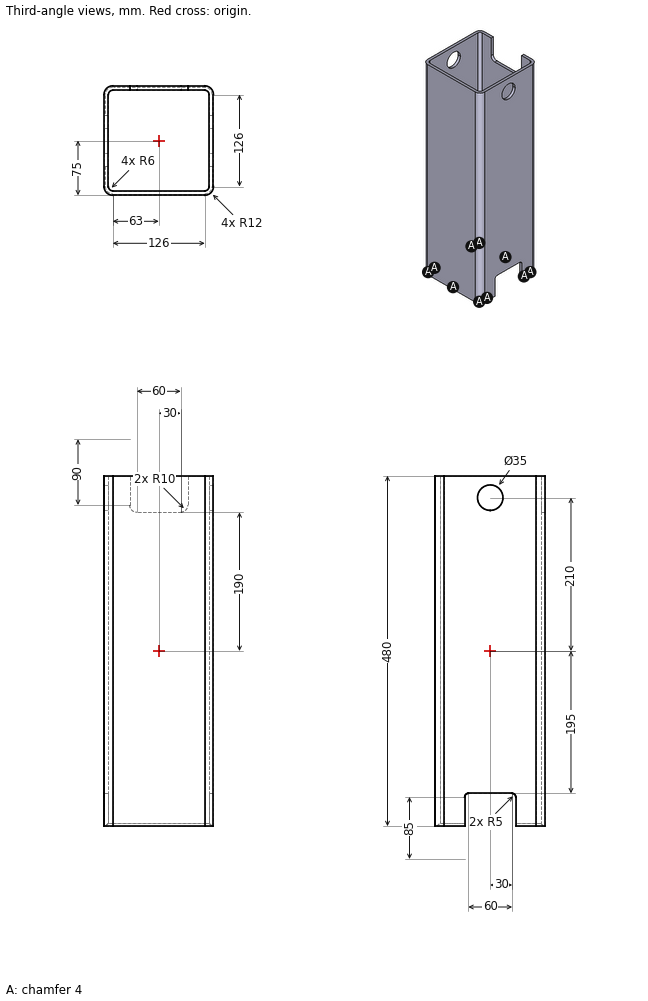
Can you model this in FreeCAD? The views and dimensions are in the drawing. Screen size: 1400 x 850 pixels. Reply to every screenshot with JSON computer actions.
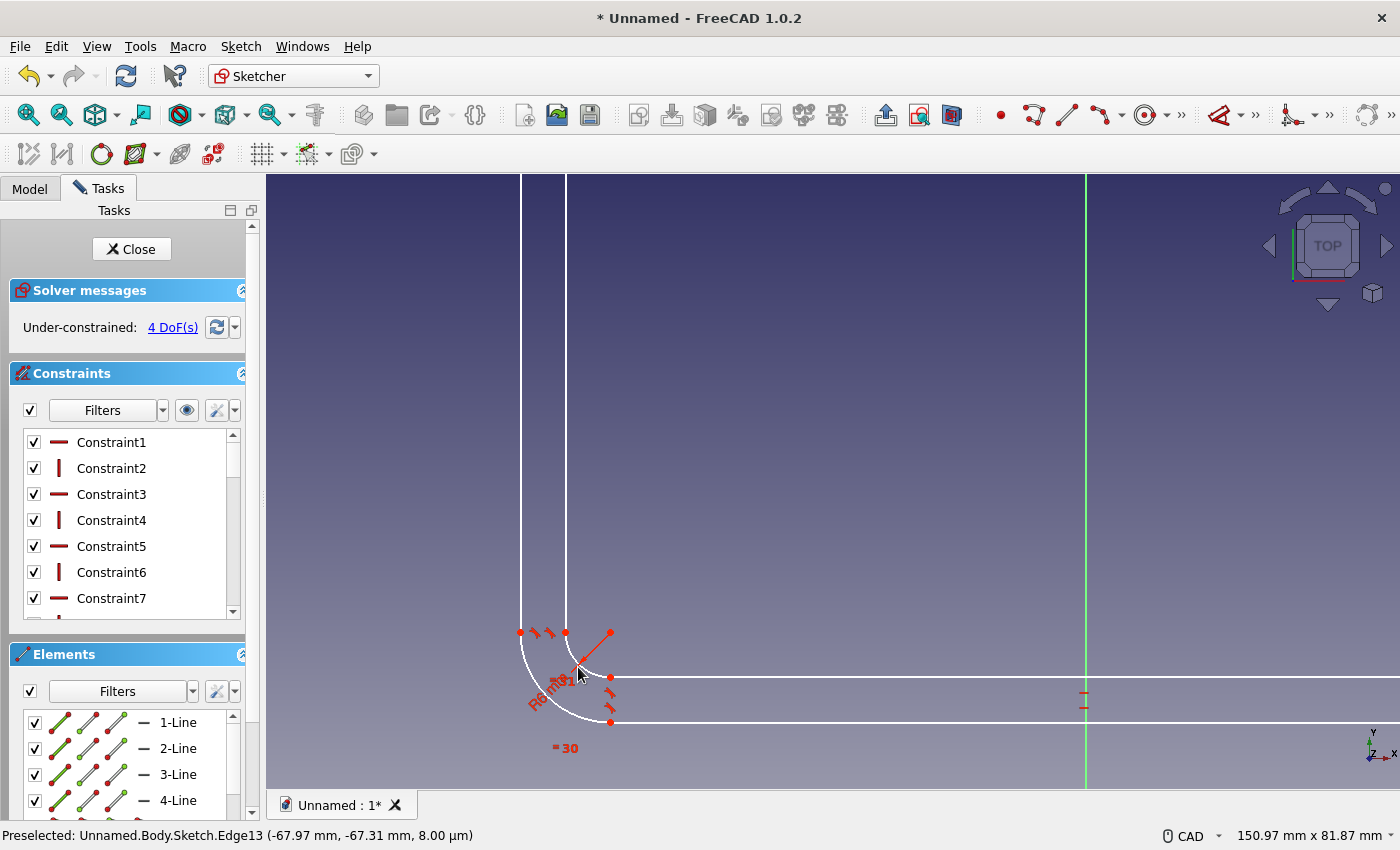
{"action": "left_click", "coordinate": [895, 723]}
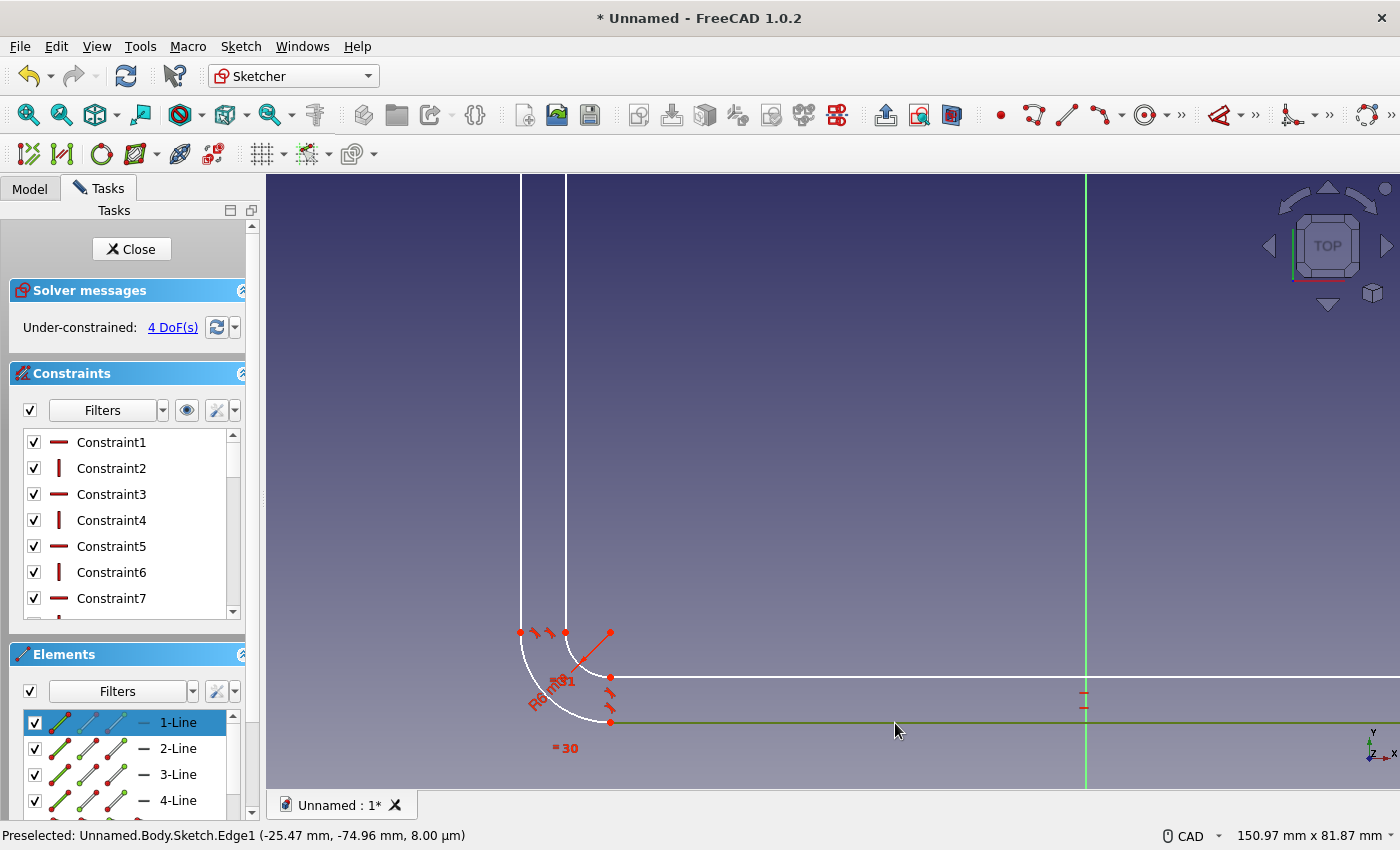
{"action": "key", "text": "l"}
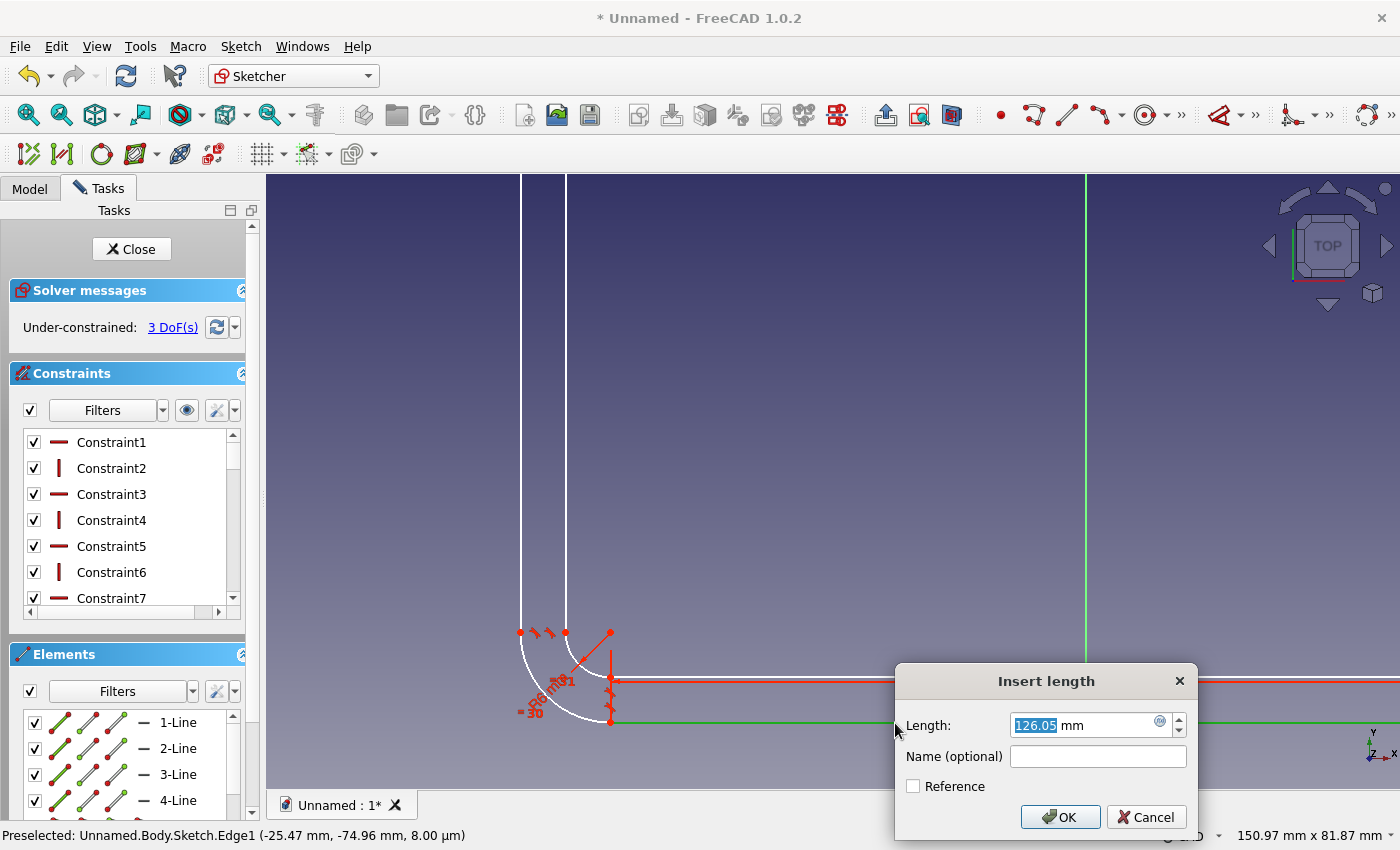
{"action": "type", "text": "126"}
{"action": "key", "text": "Return"}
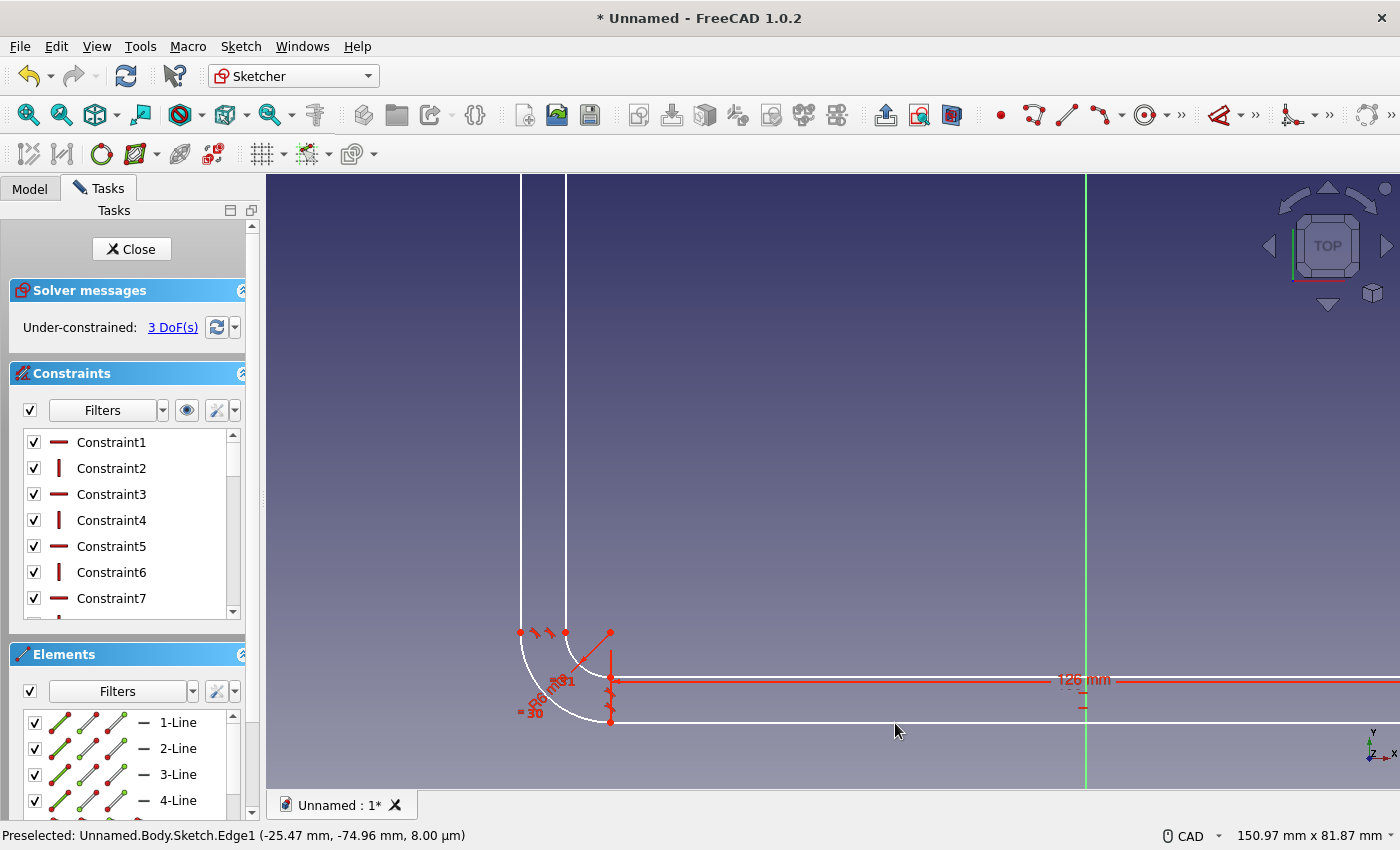
{"action": "scroll", "coordinate": [577, 669], "scroll_direction": "down", "scroll_amount": 5}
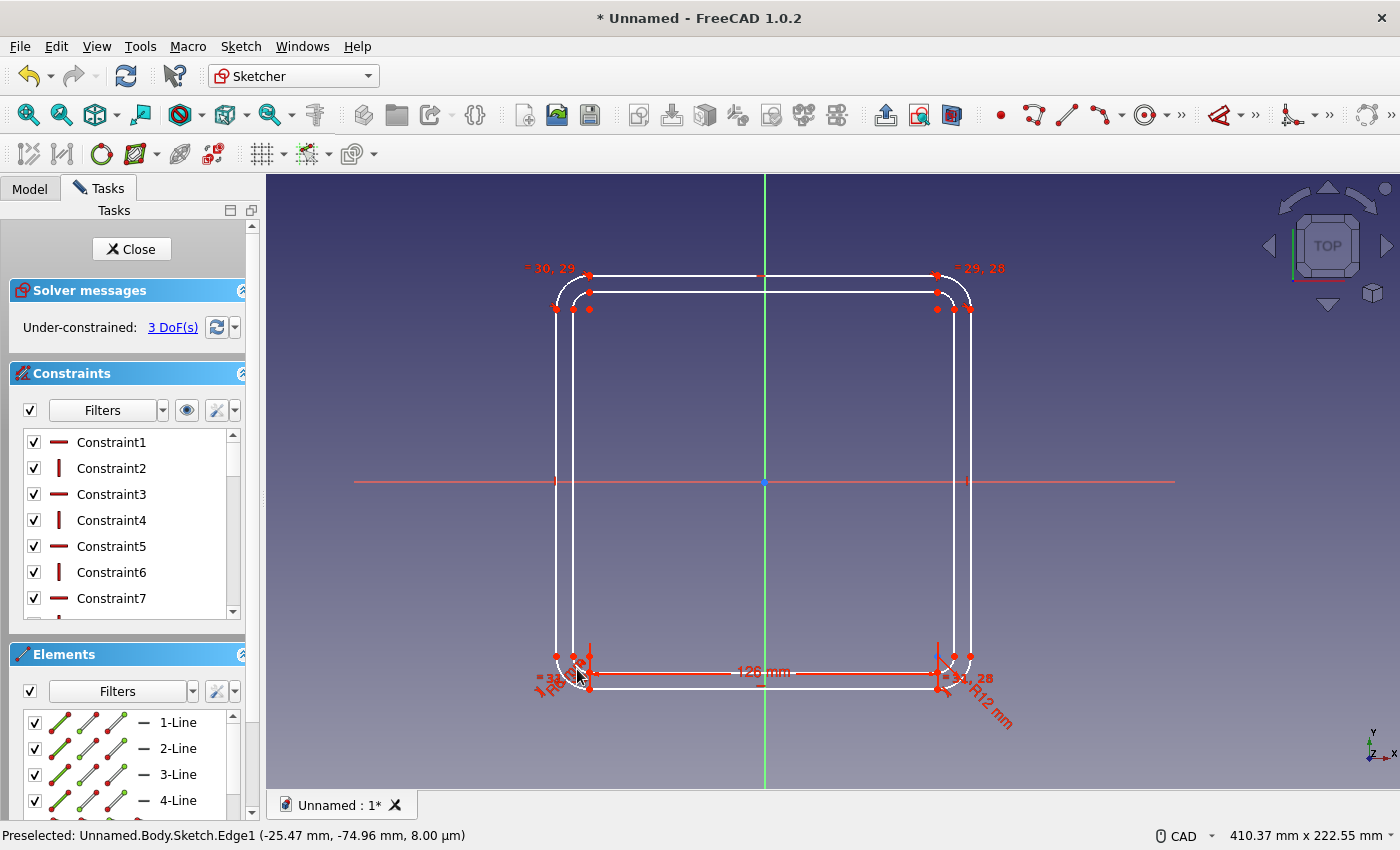
{"action": "left_click", "coordinate": [971, 552]}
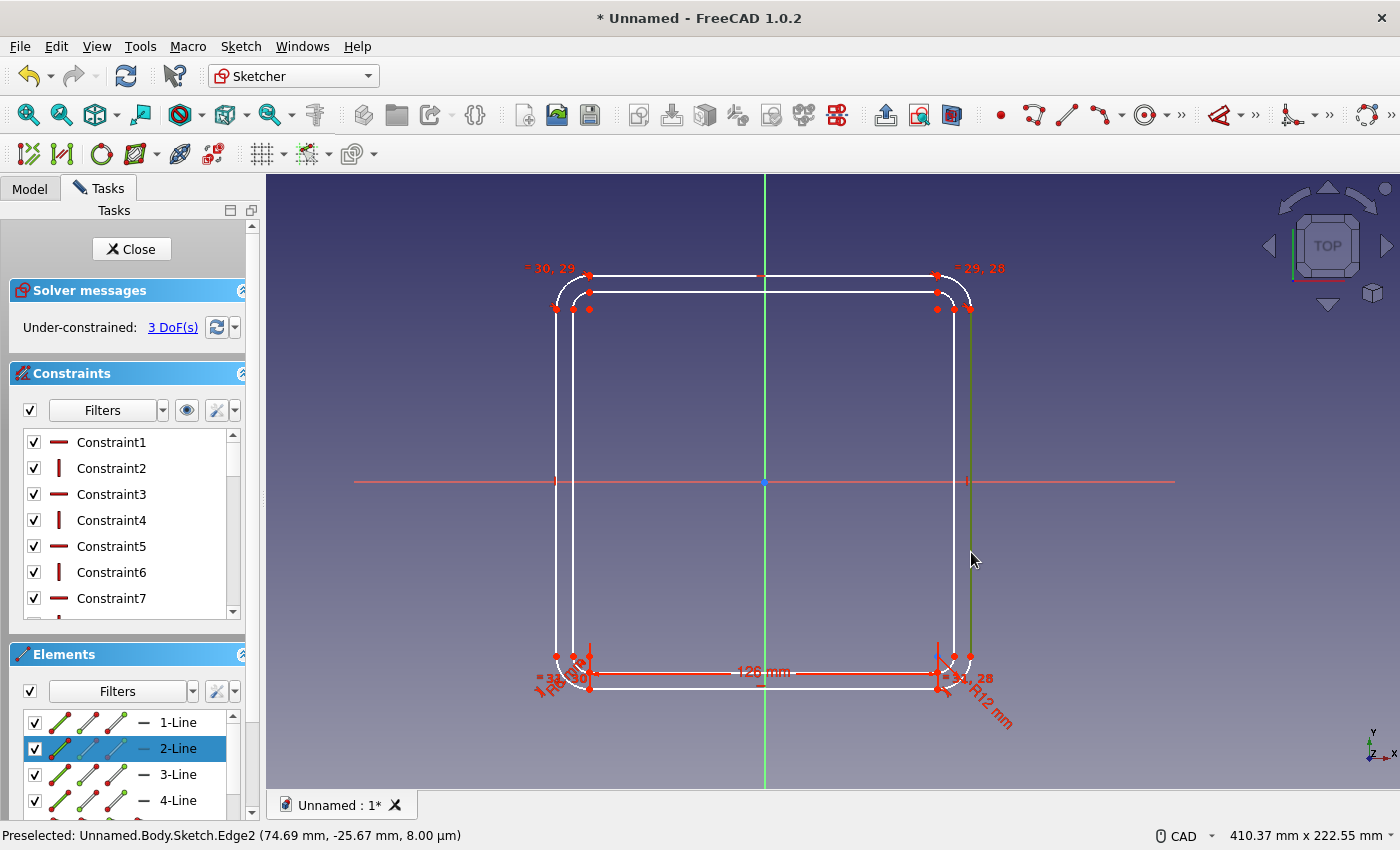
{"action": "key", "text": "i"}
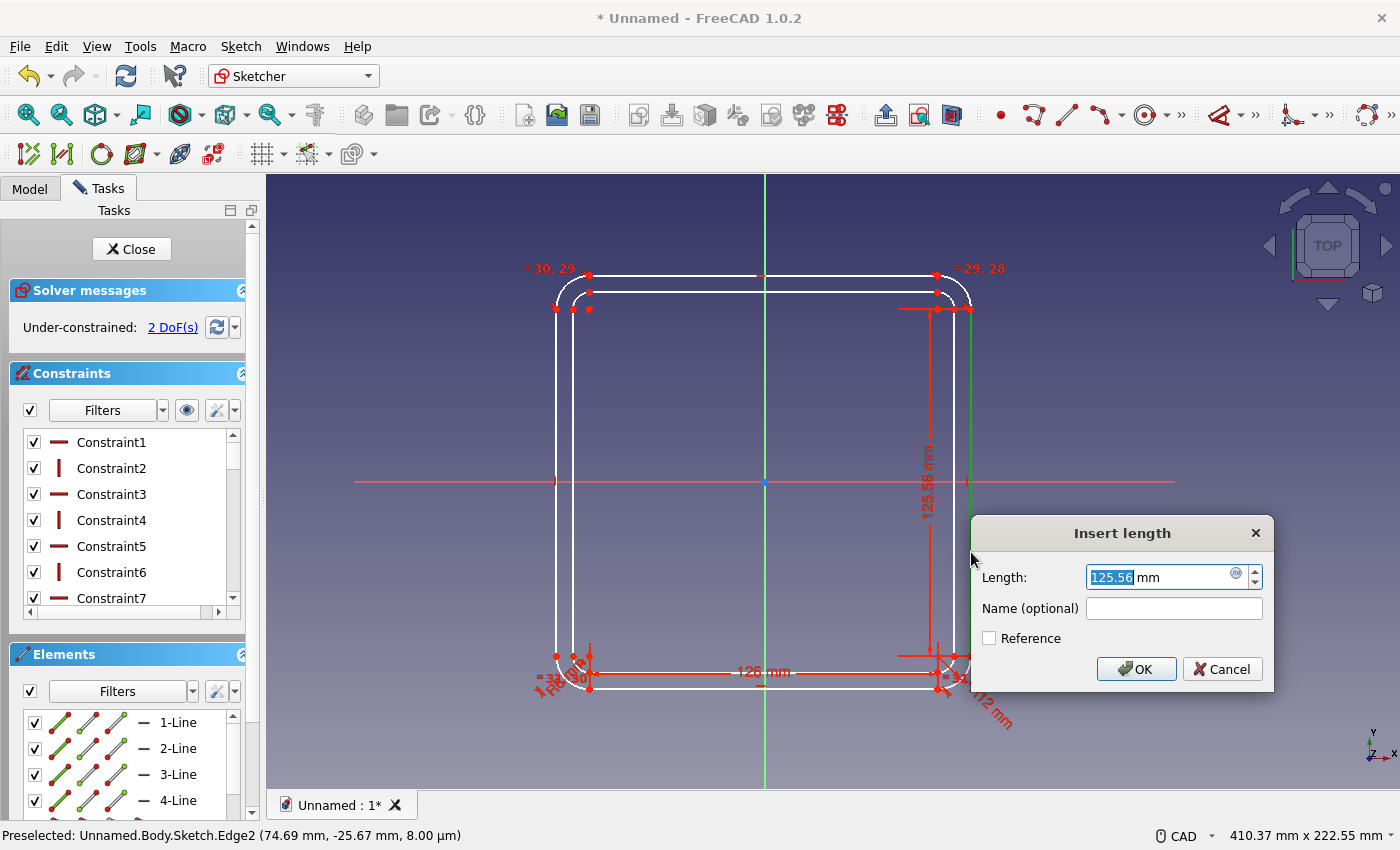
{"action": "type", "text": "126"}
{"action": "key", "text": "Return"}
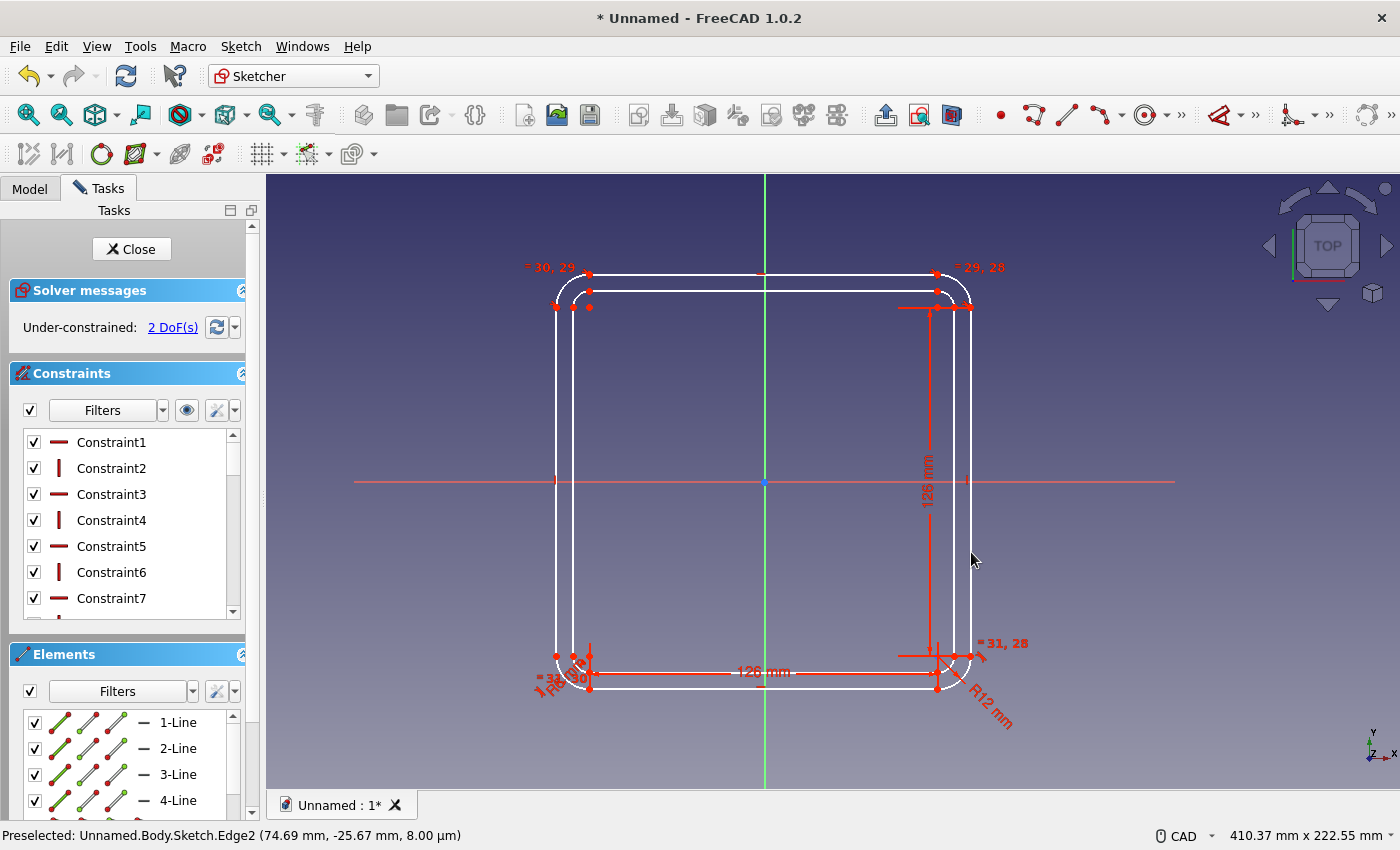
{"action": "left_click", "coordinate": [590, 689]}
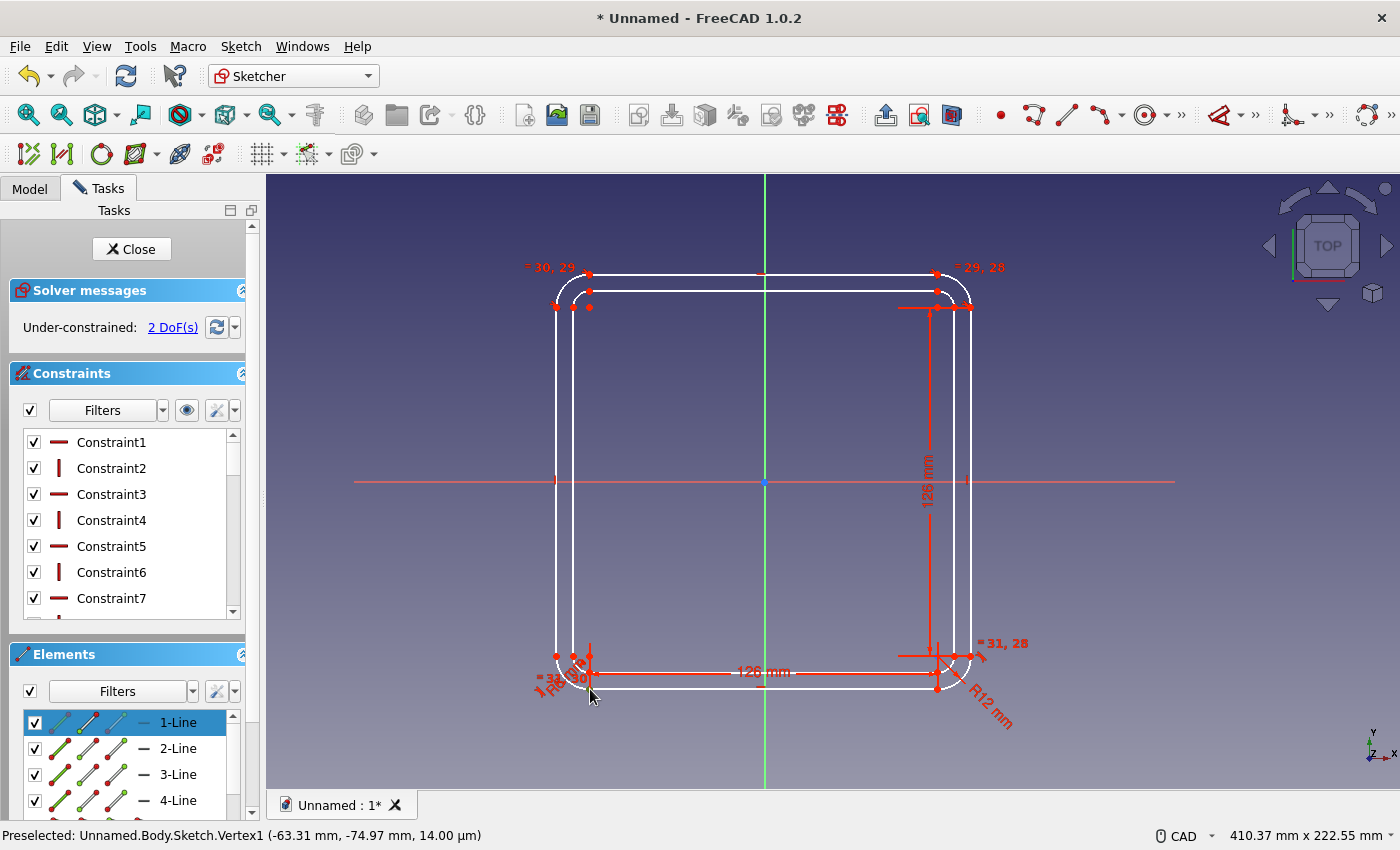
{"action": "key", "text": "l"}